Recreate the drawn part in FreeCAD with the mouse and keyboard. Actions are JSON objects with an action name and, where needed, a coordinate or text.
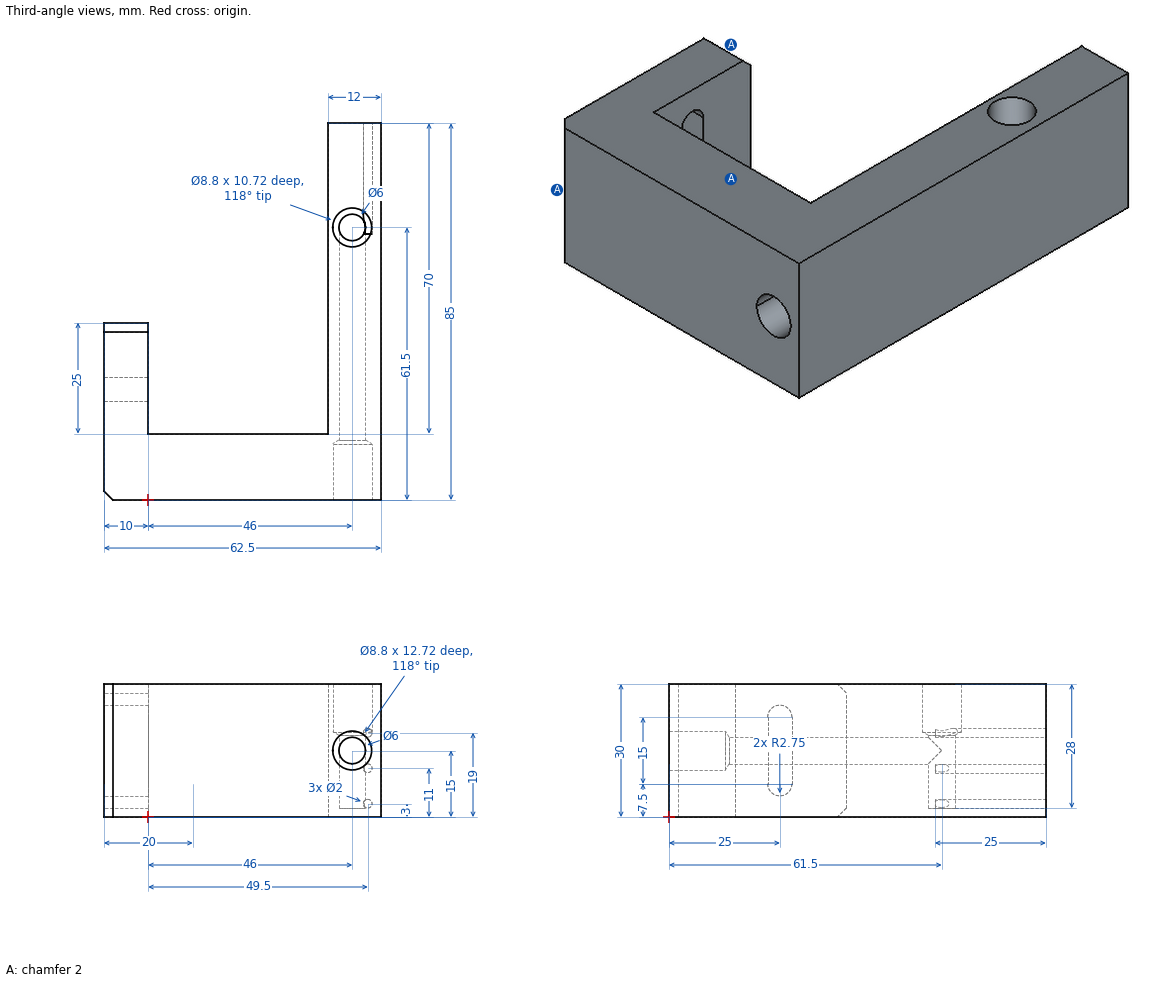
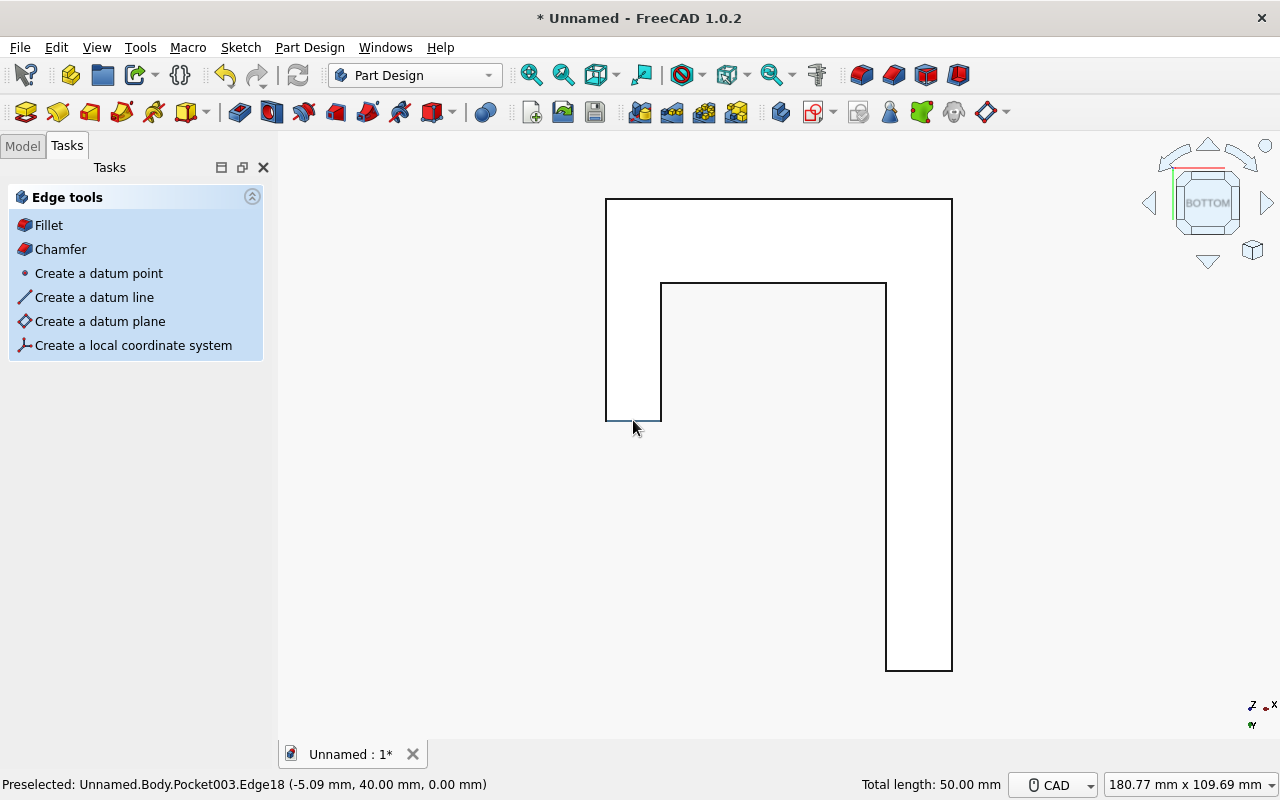
{"action": "left_click", "coordinate": [894, 76]}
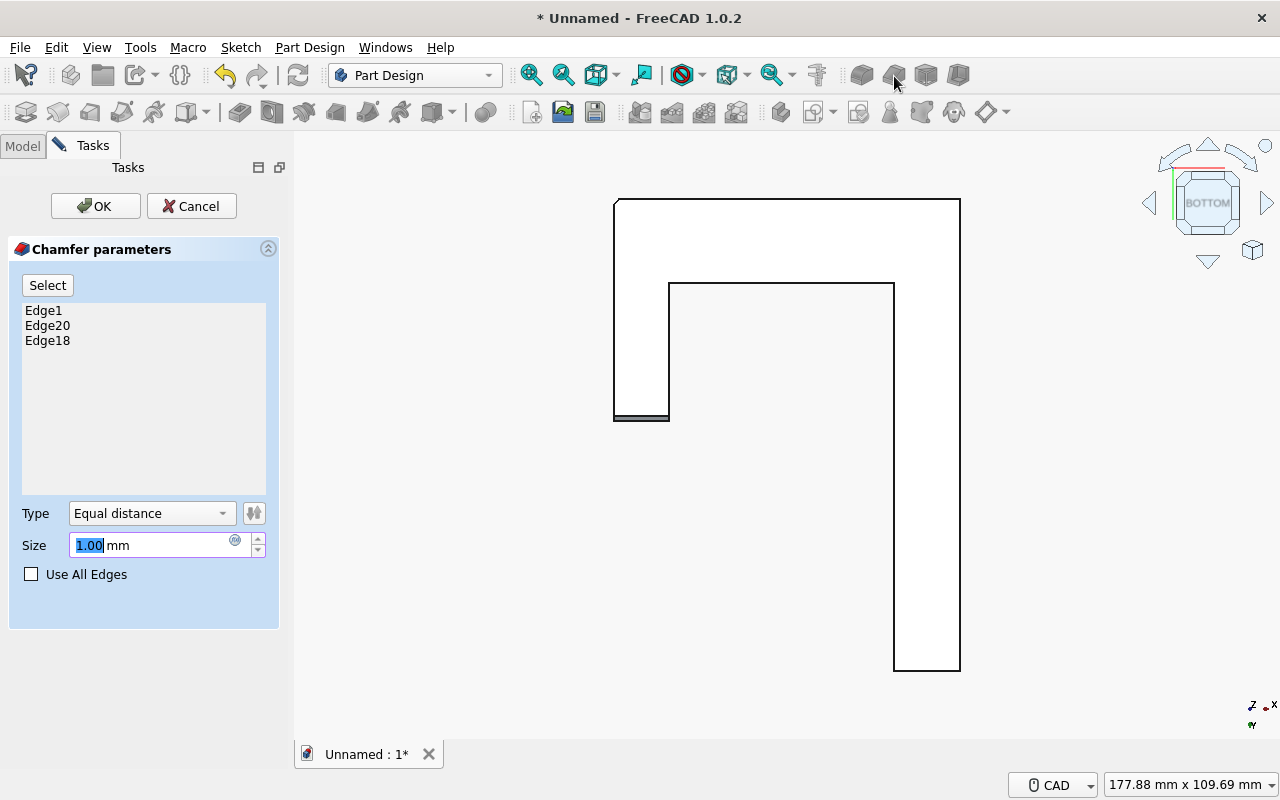
{"action": "type", "text": "2"}
{"action": "key", "text": "Tab"}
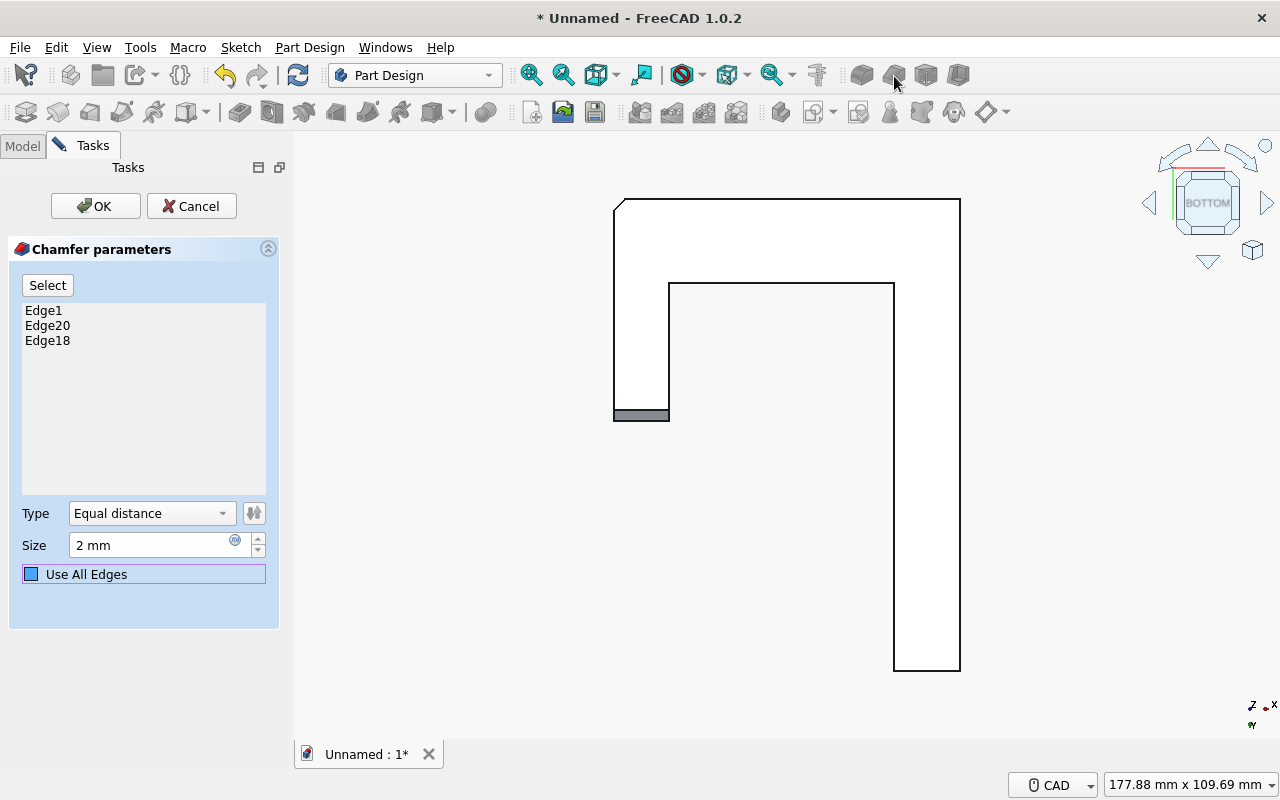
{"action": "left_click", "coordinate": [96, 206]}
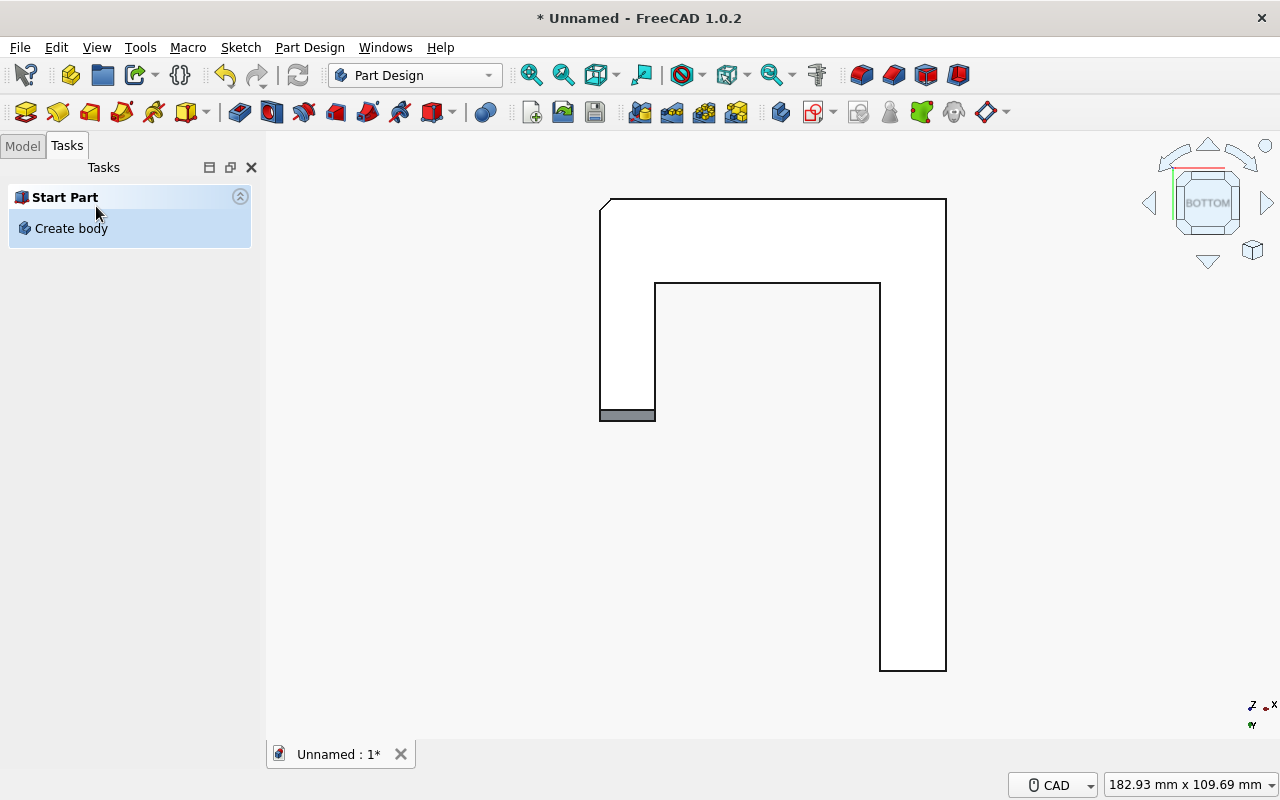
{"action": "key", "text": "0"}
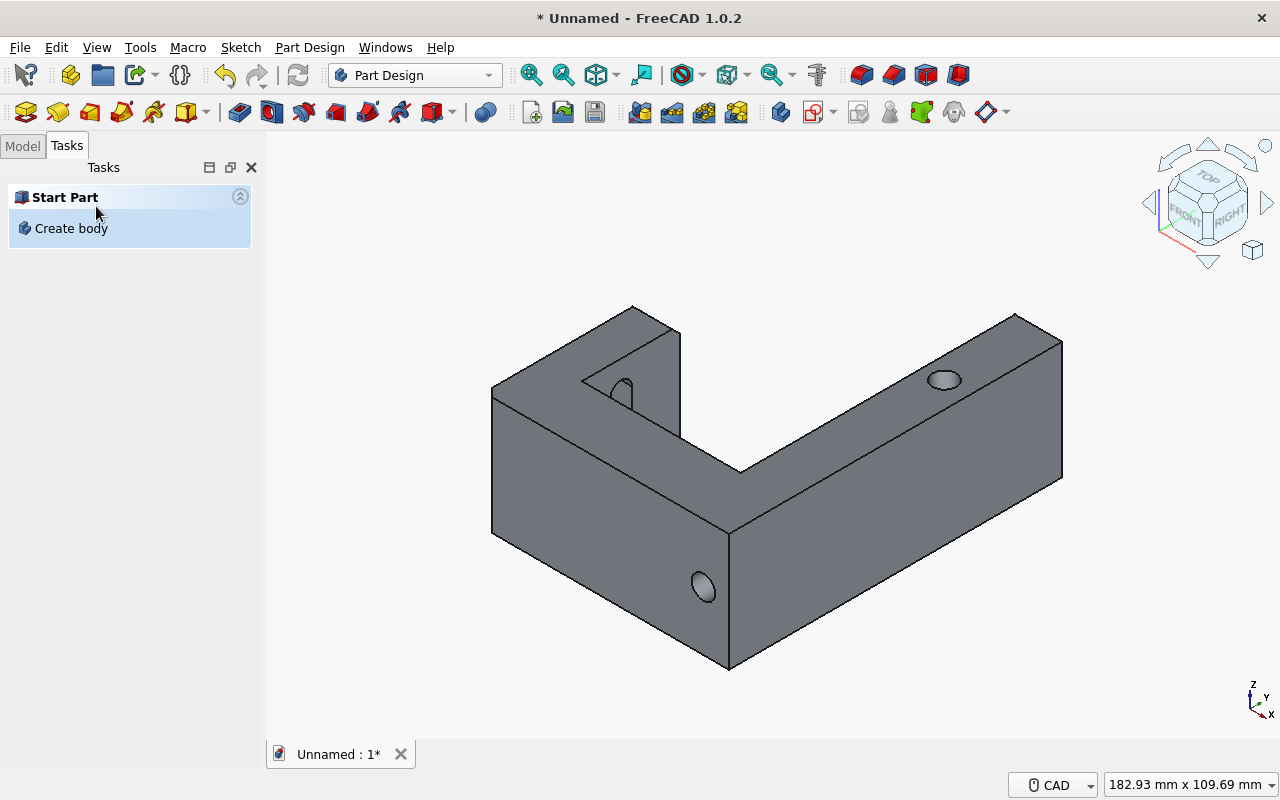
{"action": "left_click", "coordinate": [610, 532]}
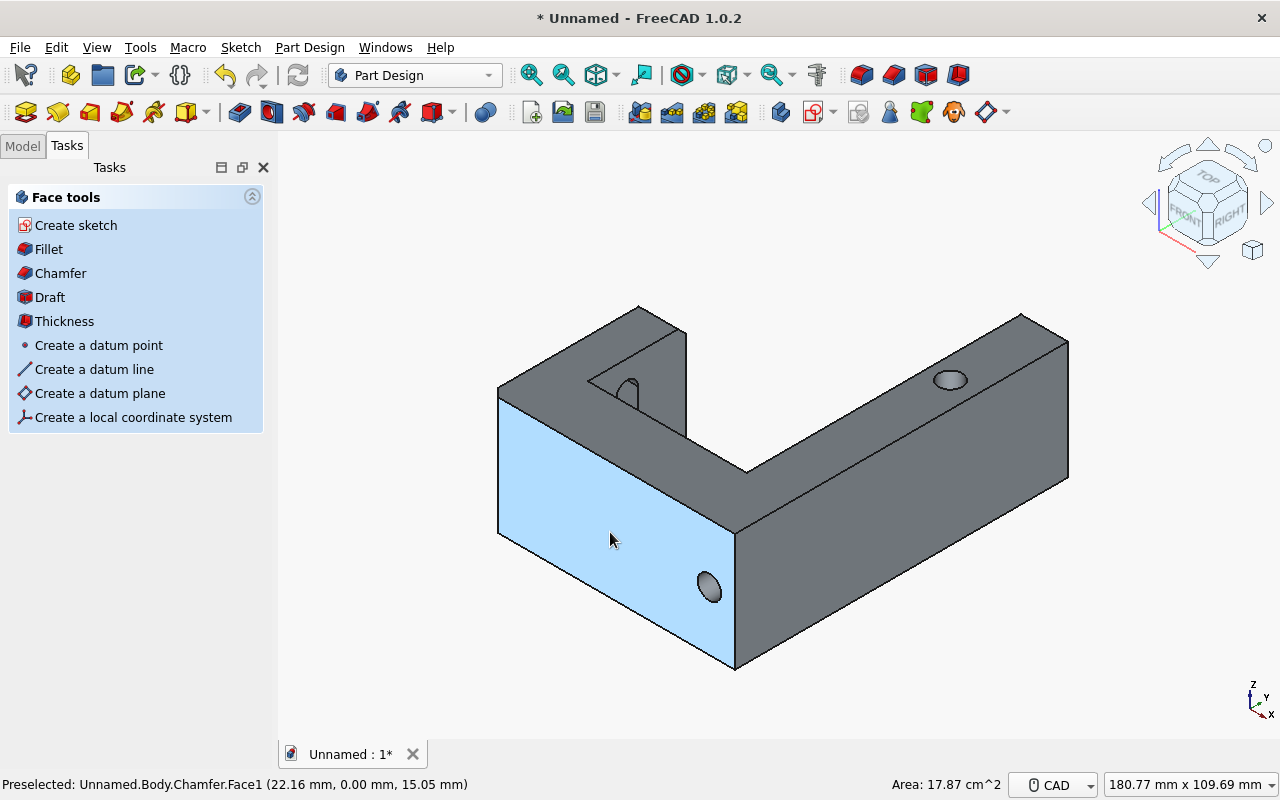
{"action": "left_click", "coordinate": [814, 112]}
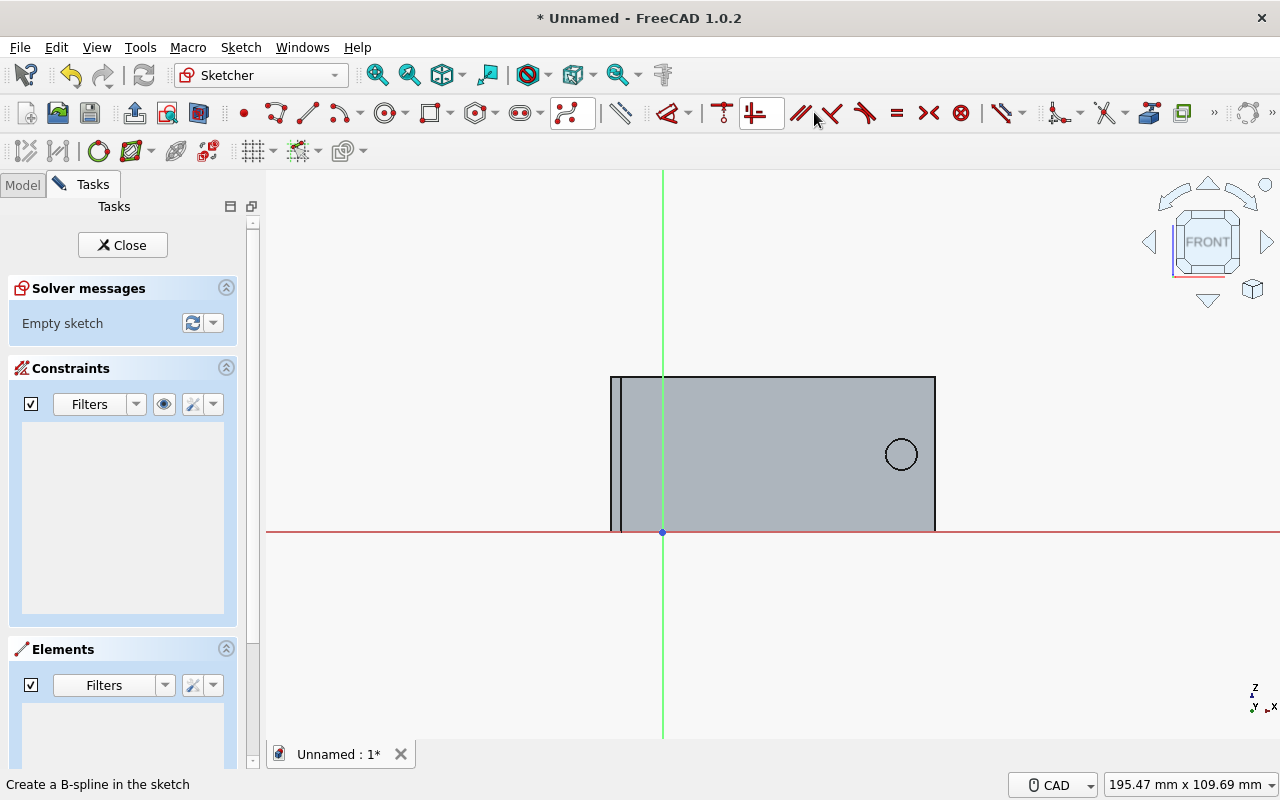
{"action": "scroll", "coordinate": [932, 454], "scroll_direction": "up", "scroll_amount": 10}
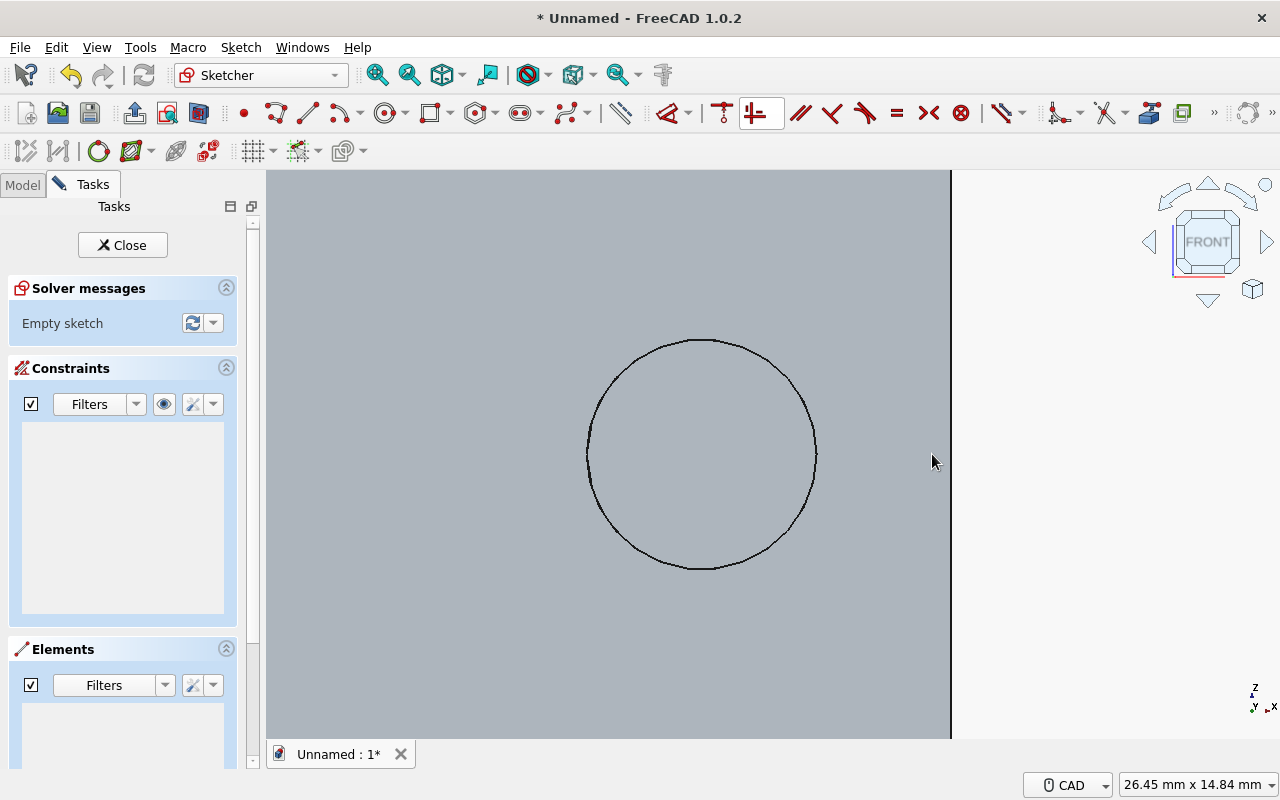
{"action": "key", "text": "g c"}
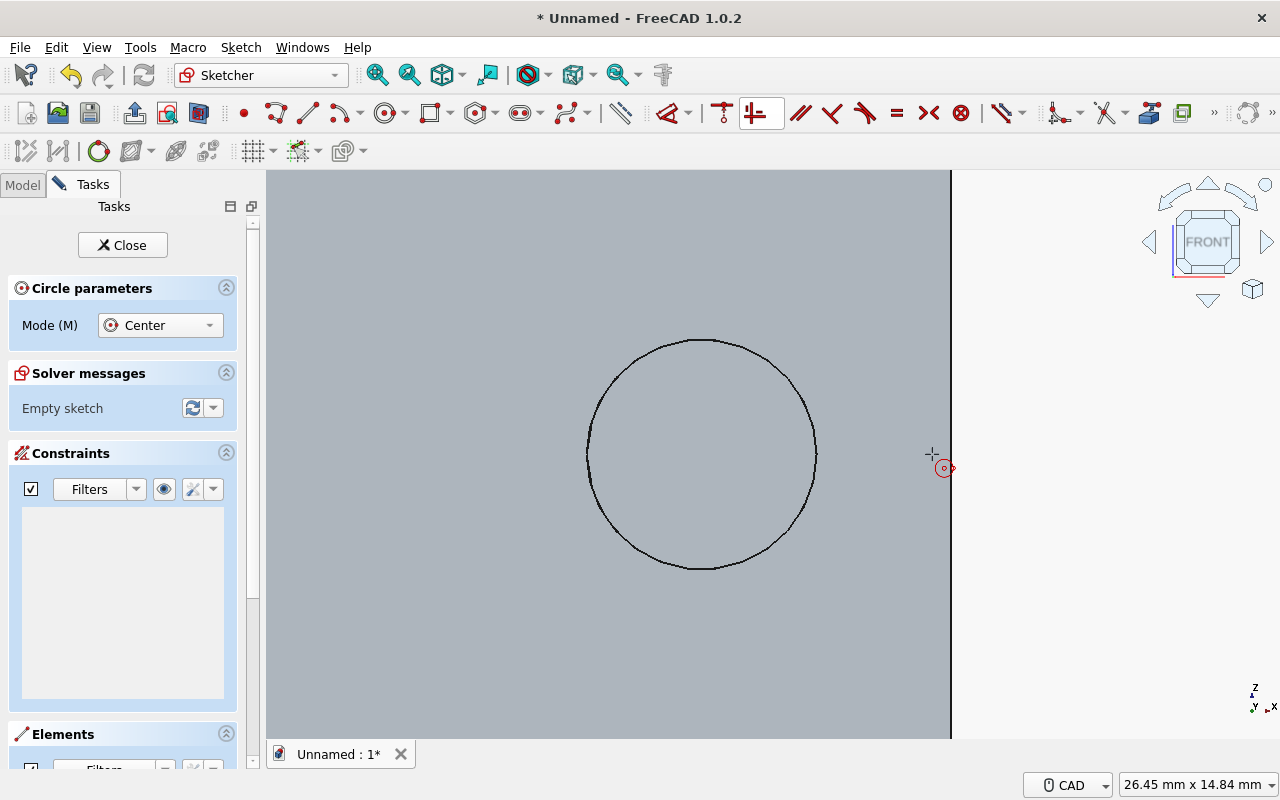
{"action": "left_click", "coordinate": [702, 454]}
{"action": "mouse_move", "coordinate": [821, 335]}